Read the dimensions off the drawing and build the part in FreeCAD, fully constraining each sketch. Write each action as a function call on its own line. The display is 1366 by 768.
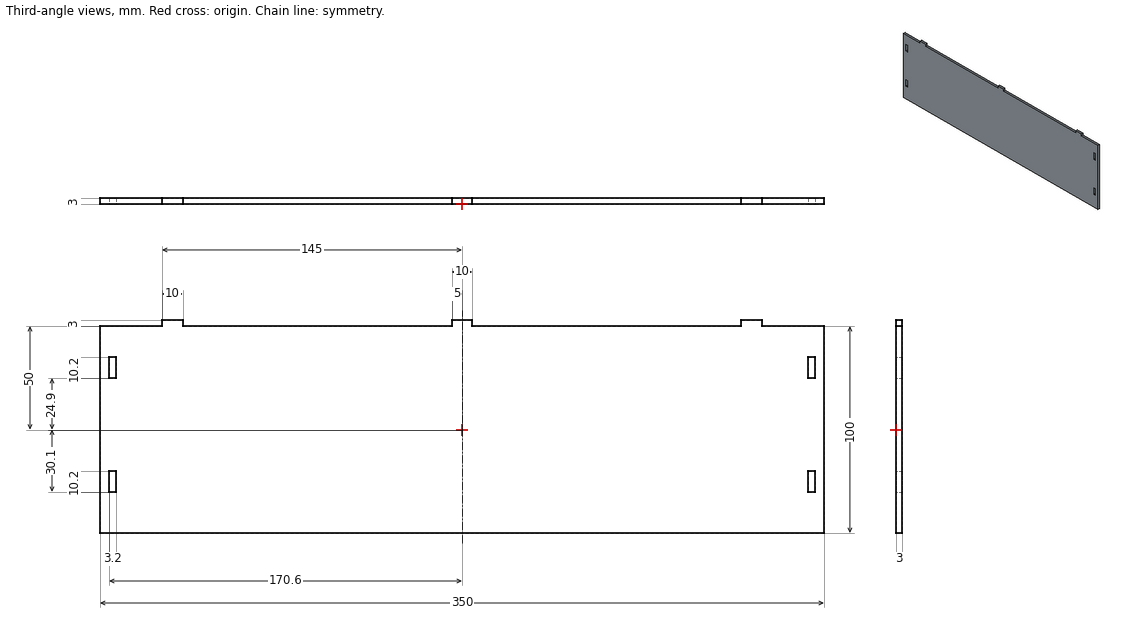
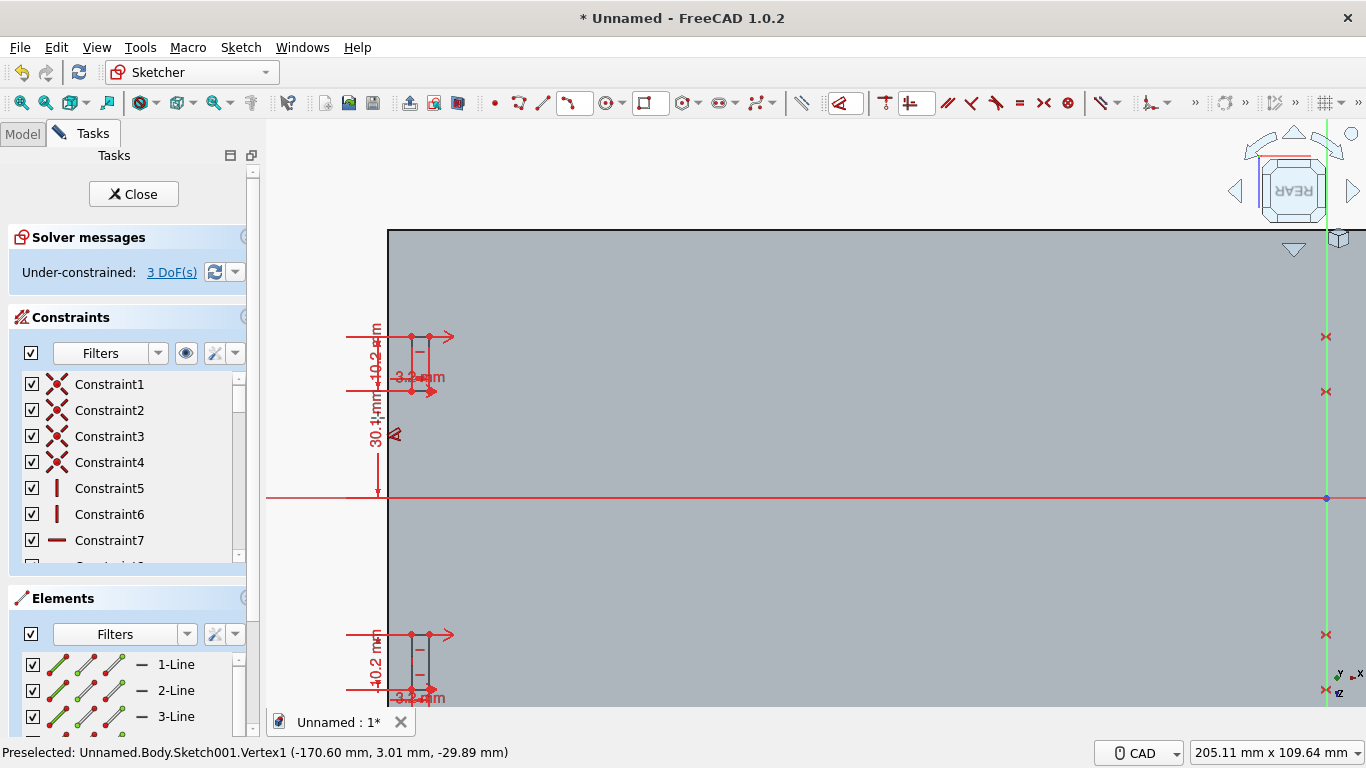
click(412, 635)
click(378, 567)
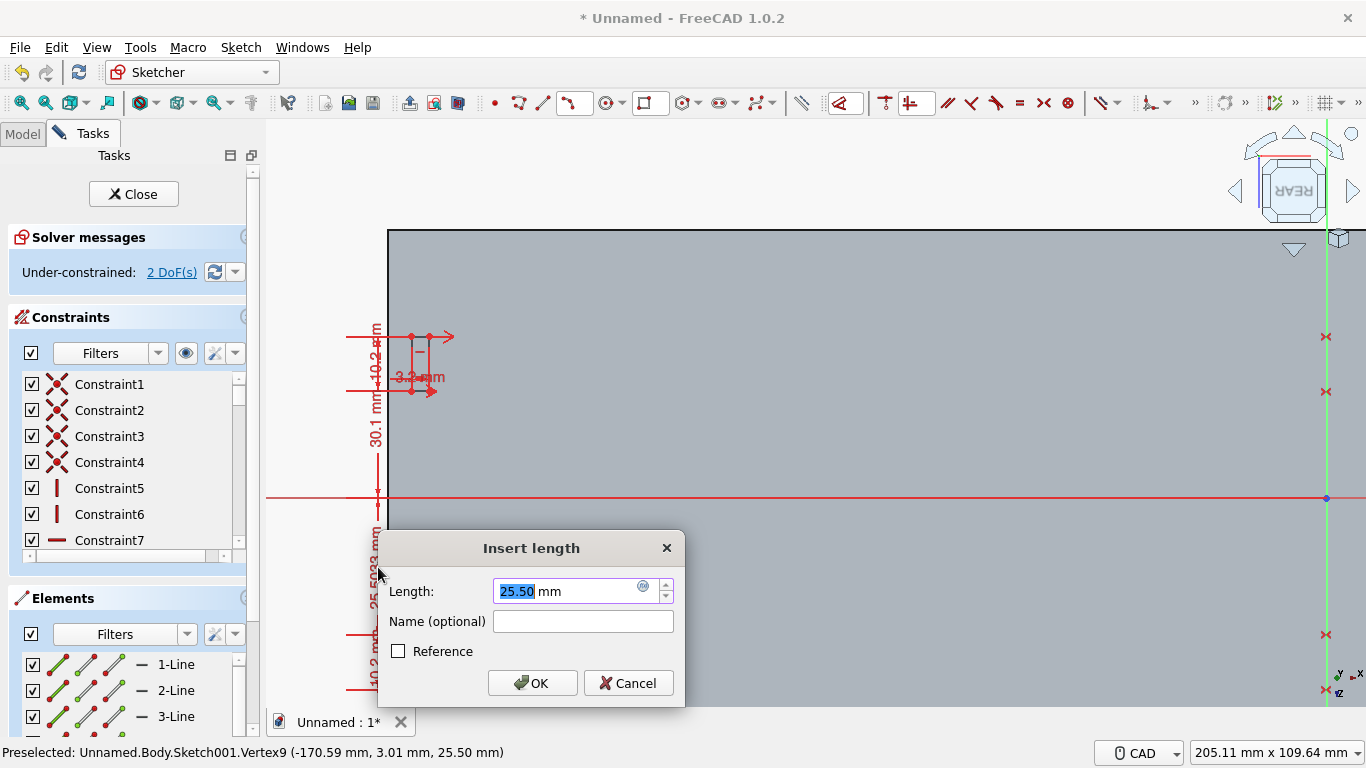
text(24.9)
key(Return)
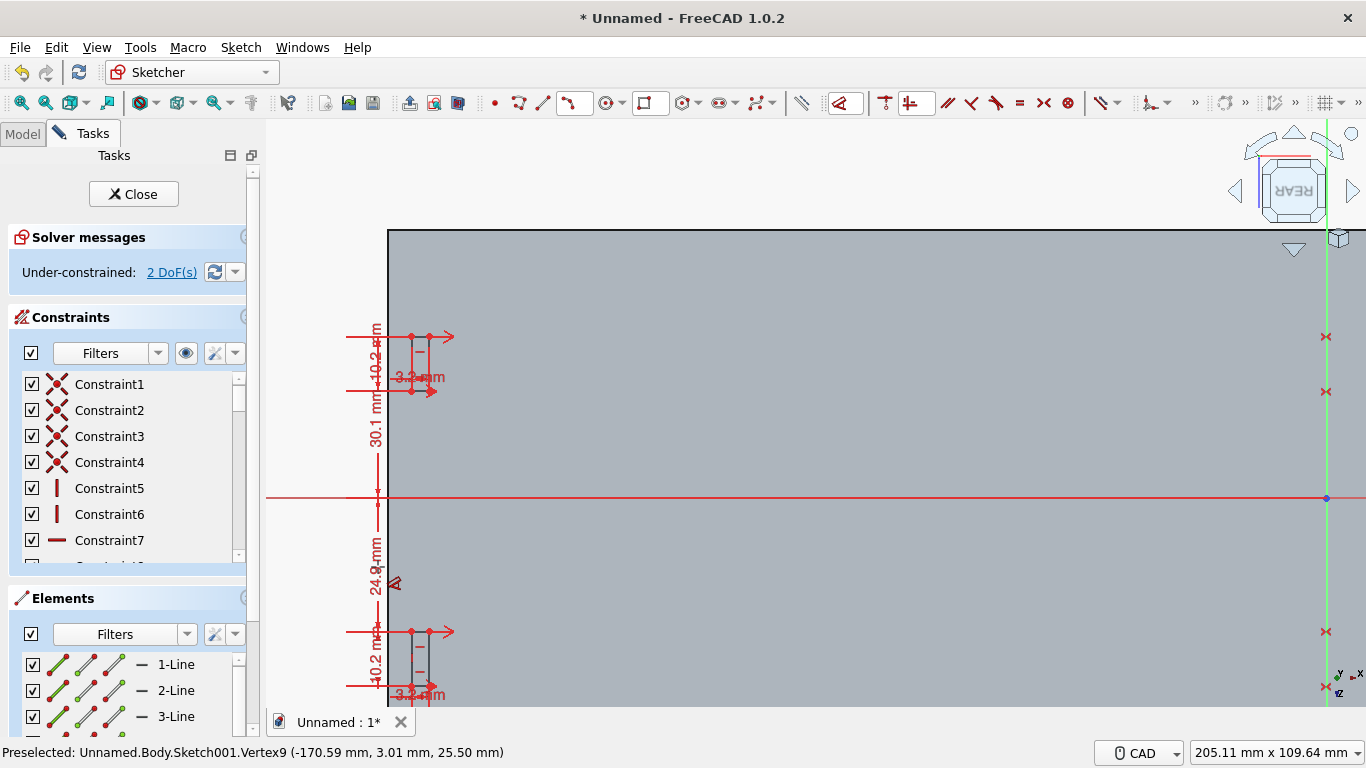
click(412, 337)
click(806, 303)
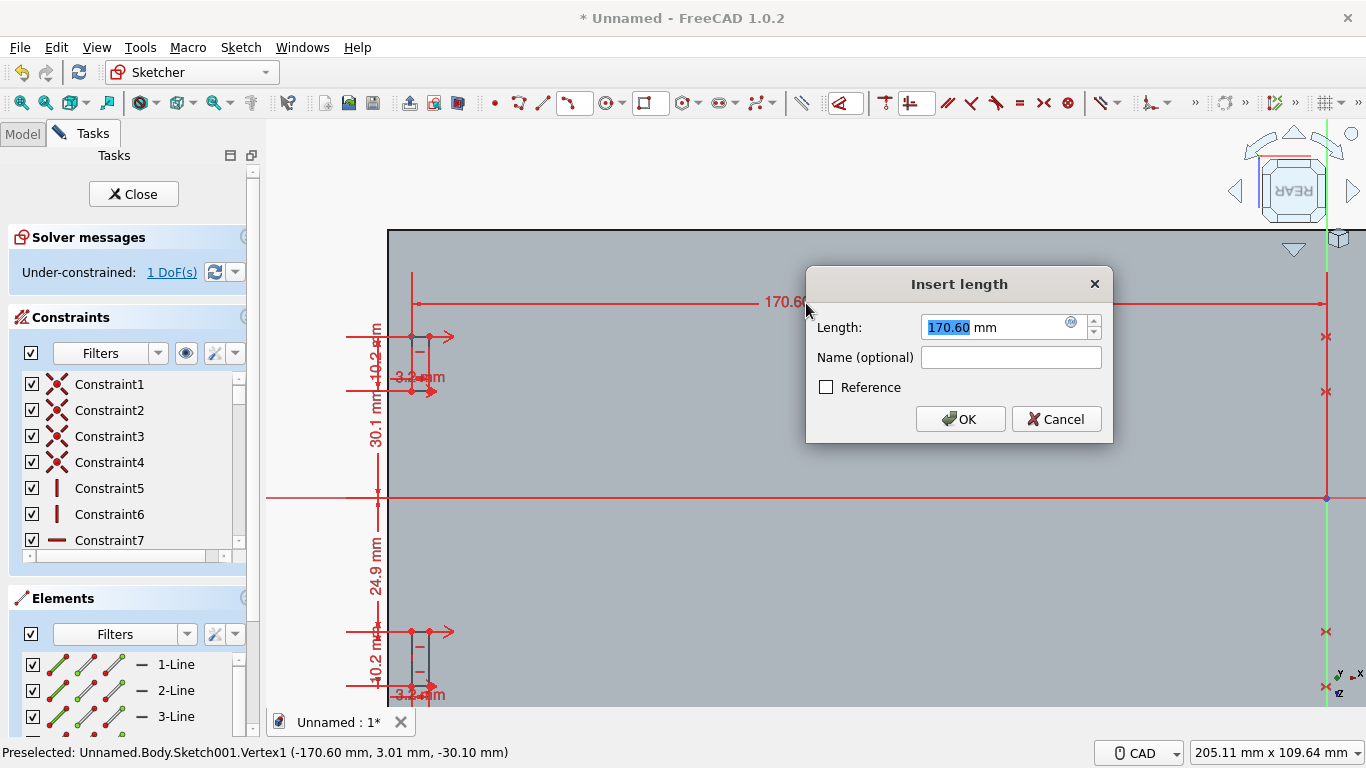
text(170.6)
key(Return)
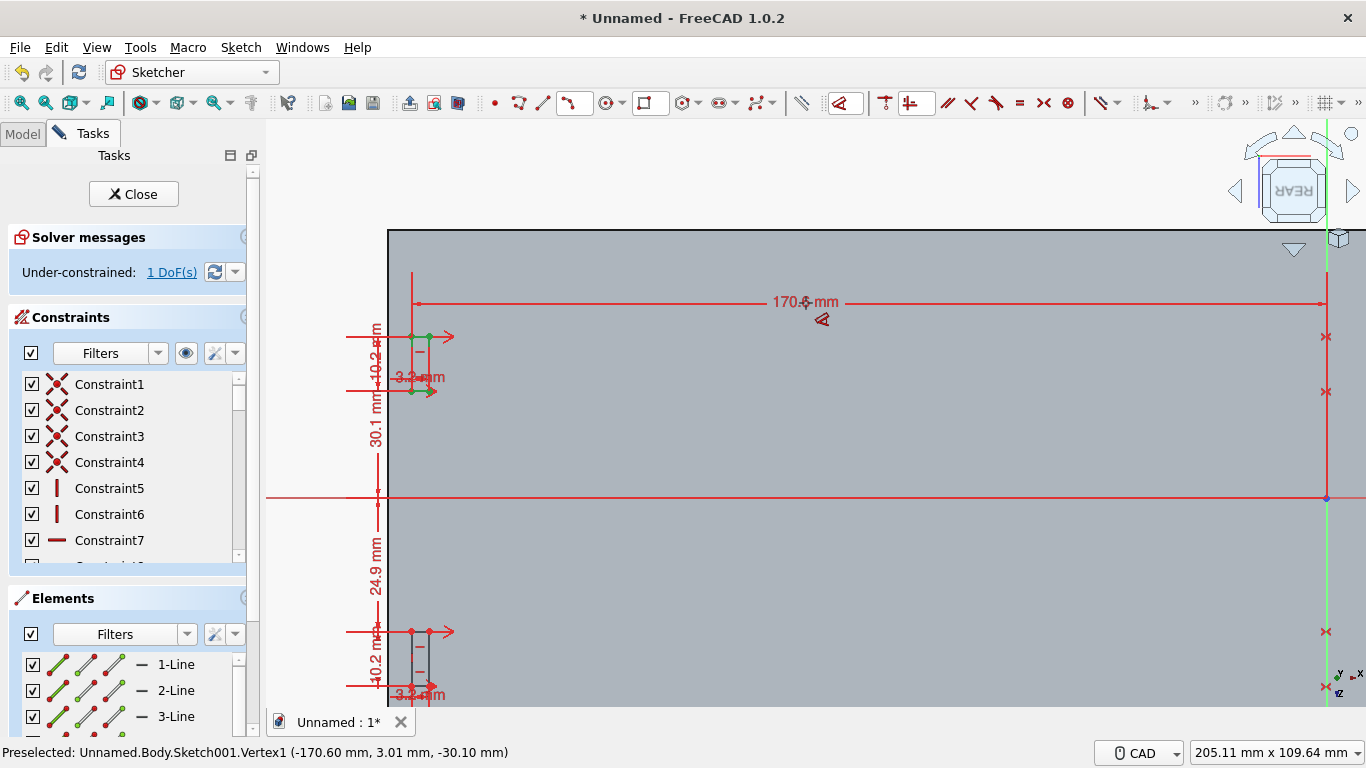
click(412, 632)
click(806, 666)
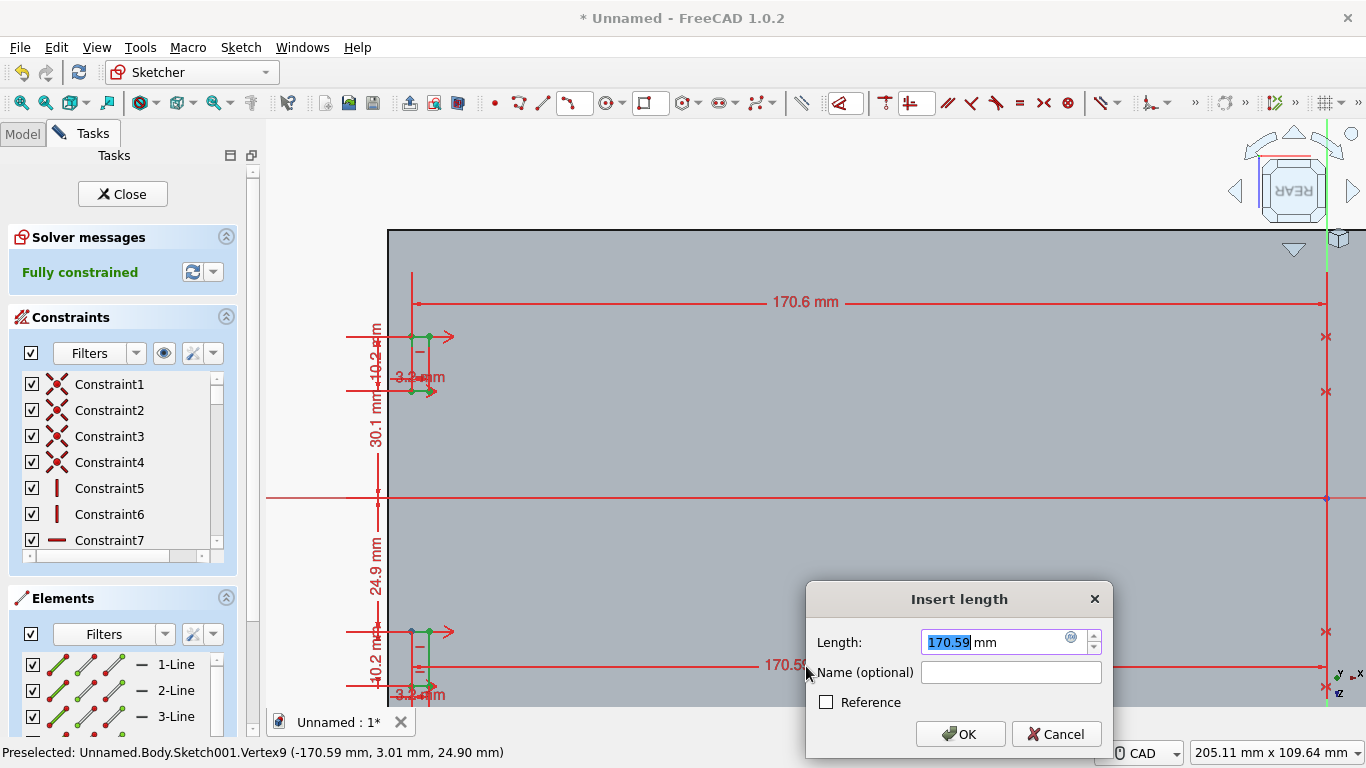
text(170.6)
key(Return)
key(Escape)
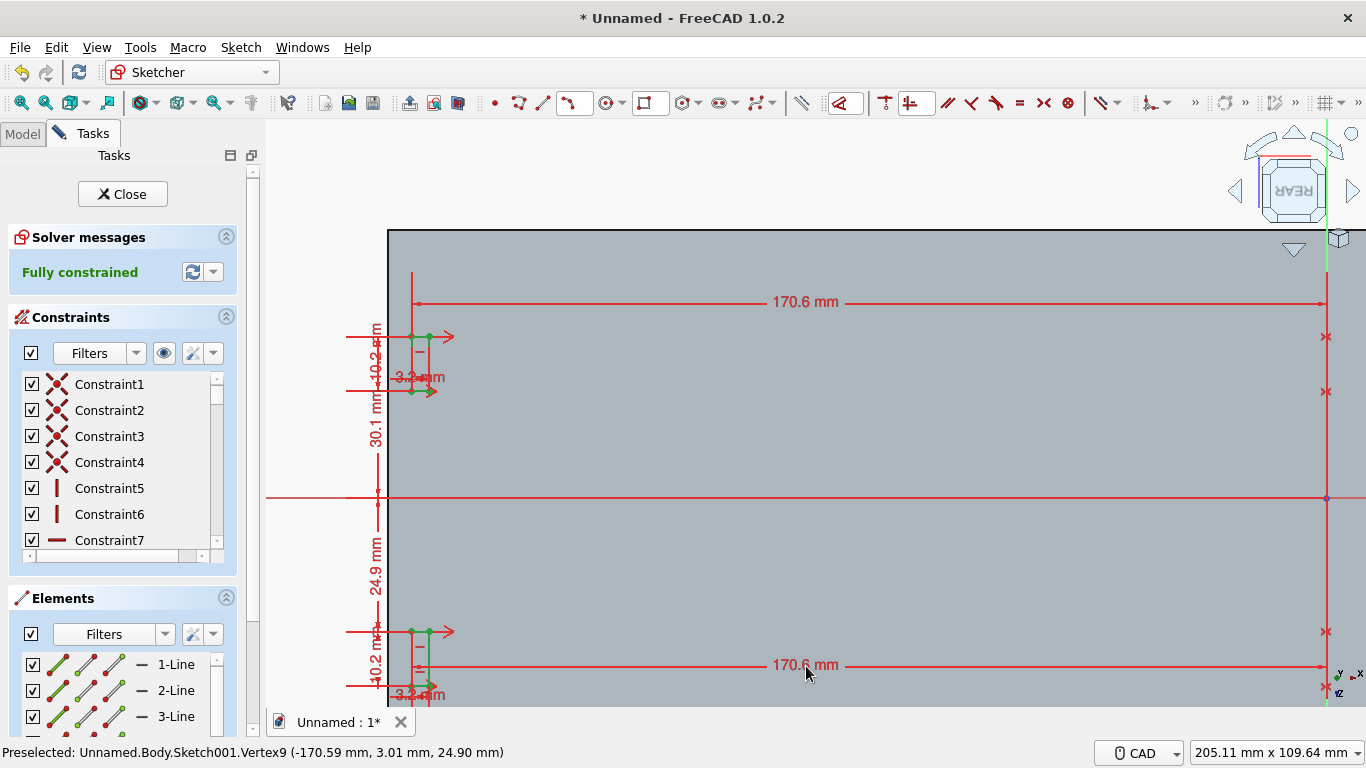
click(123, 194)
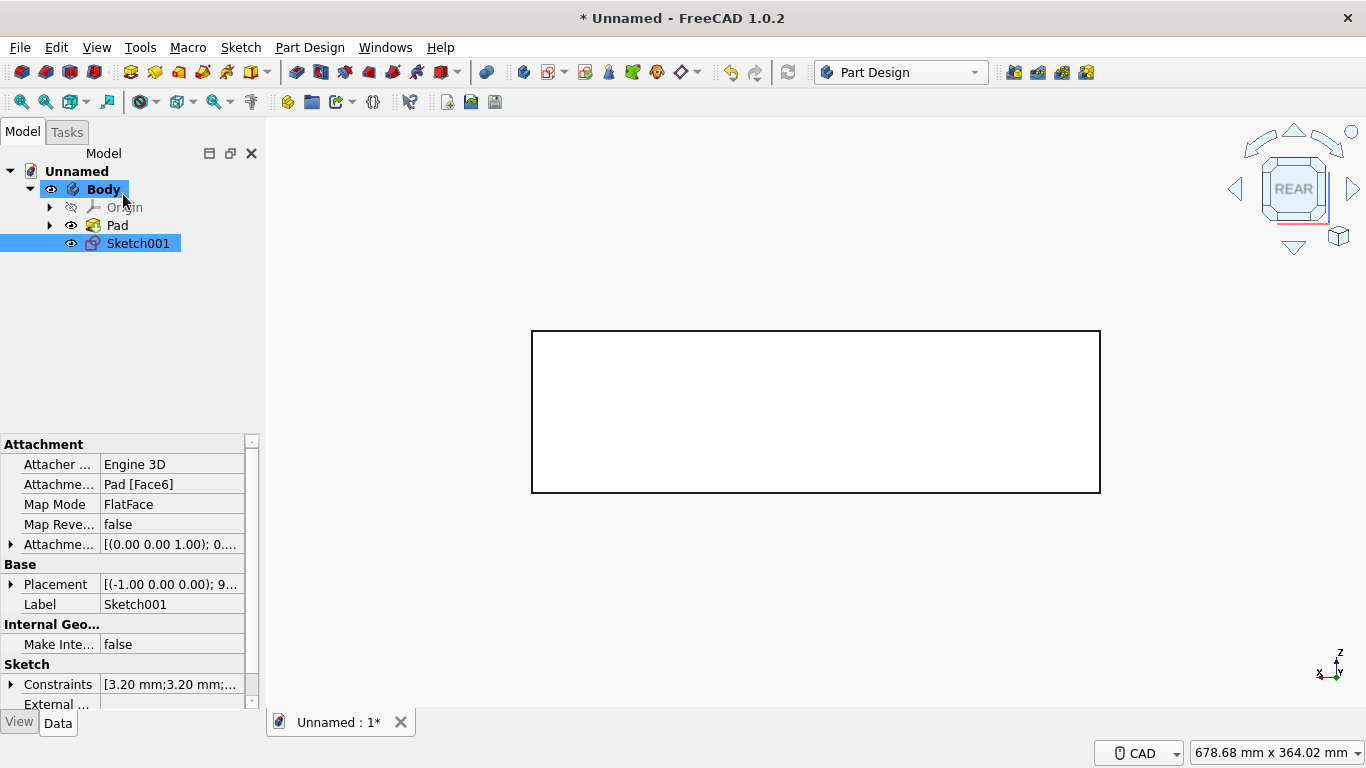
click(298, 72)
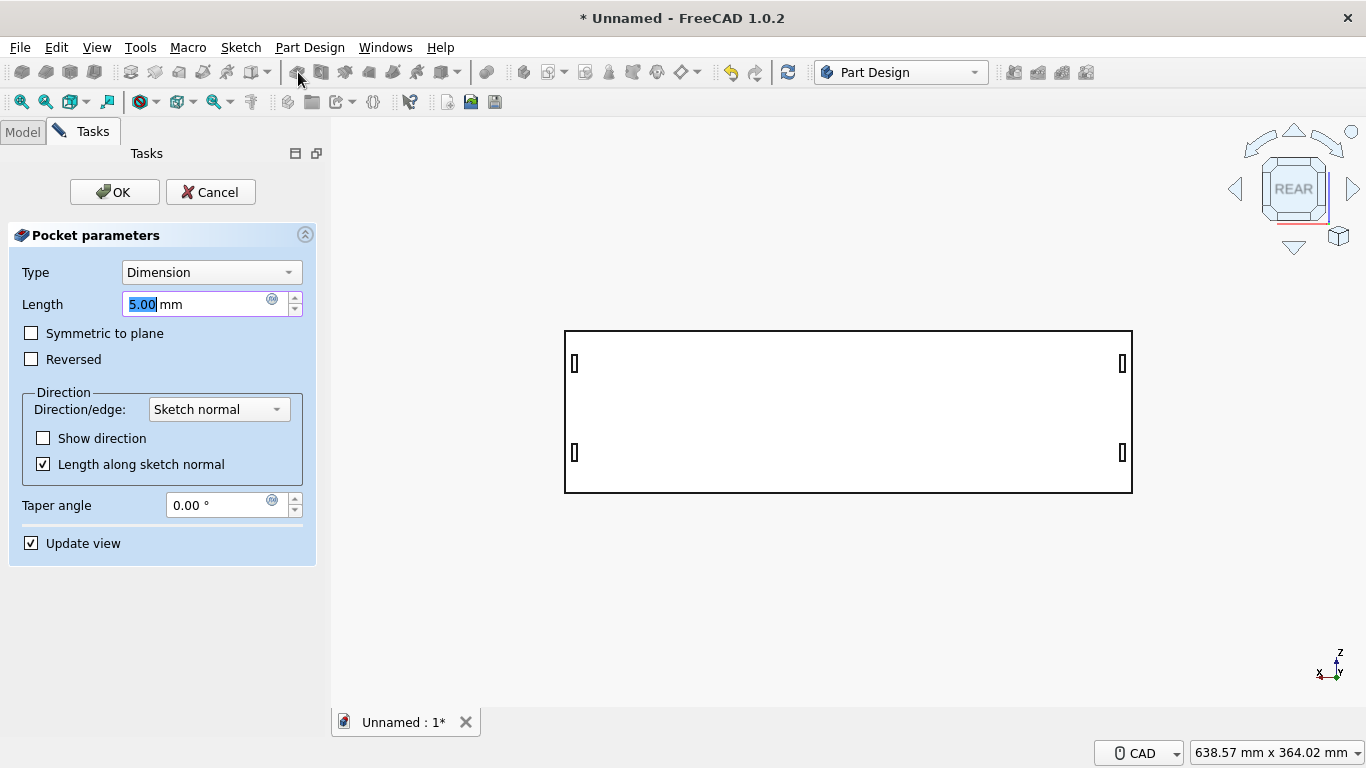
click(212, 272)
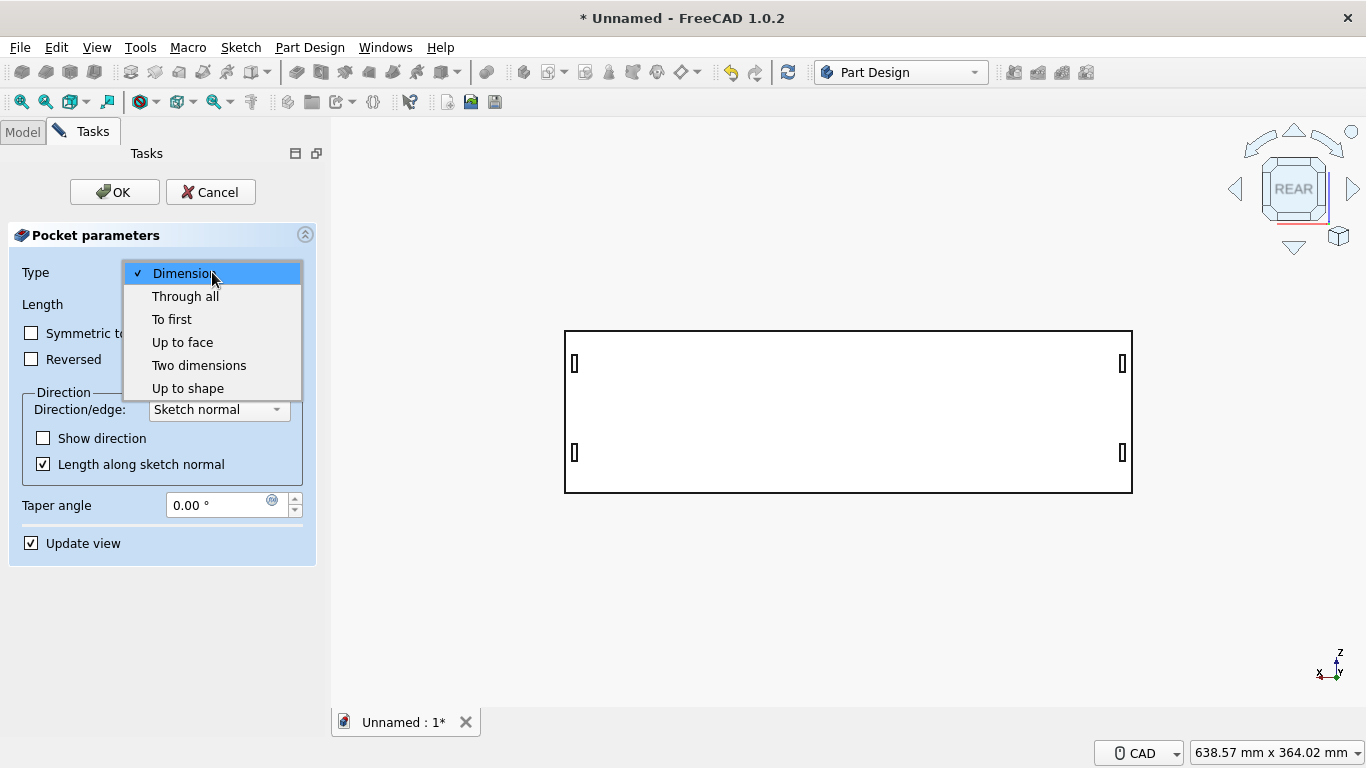
click(212, 296)